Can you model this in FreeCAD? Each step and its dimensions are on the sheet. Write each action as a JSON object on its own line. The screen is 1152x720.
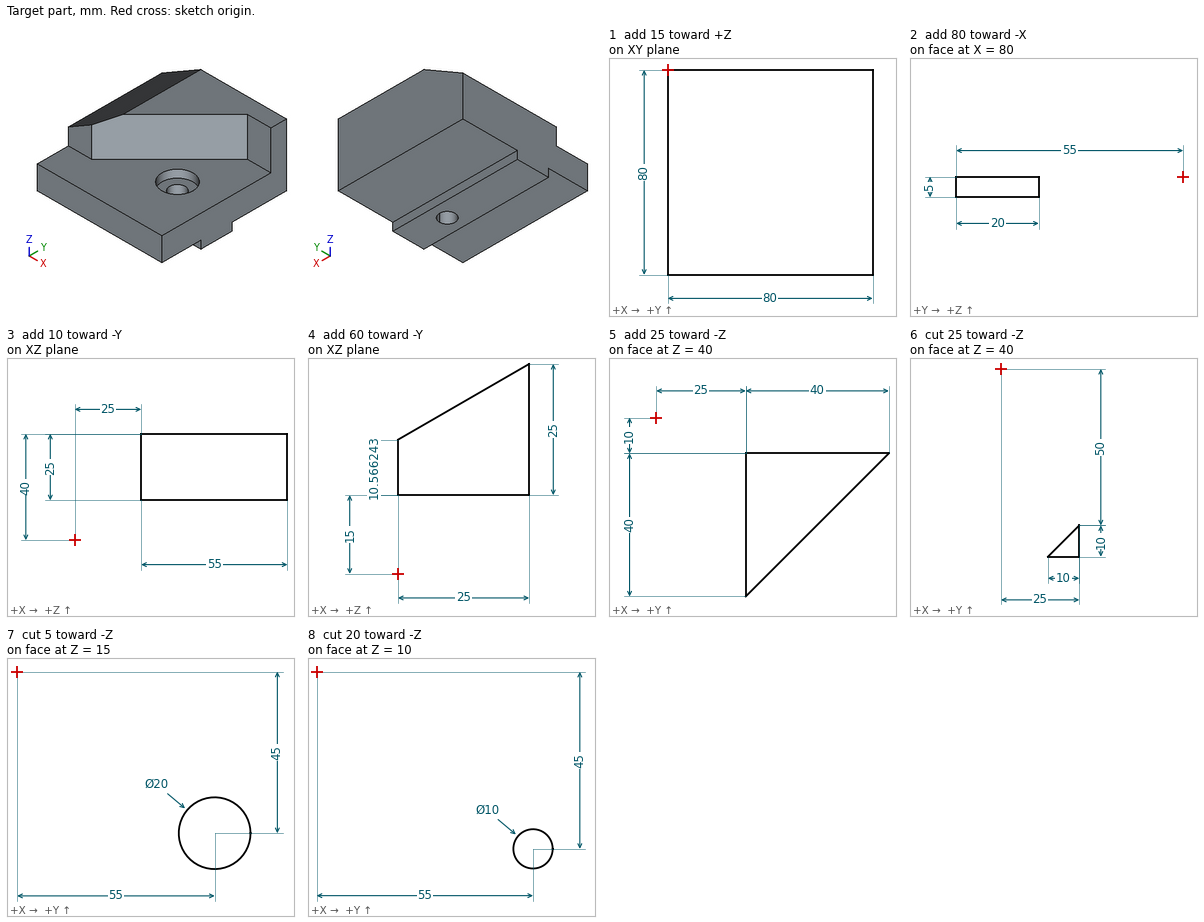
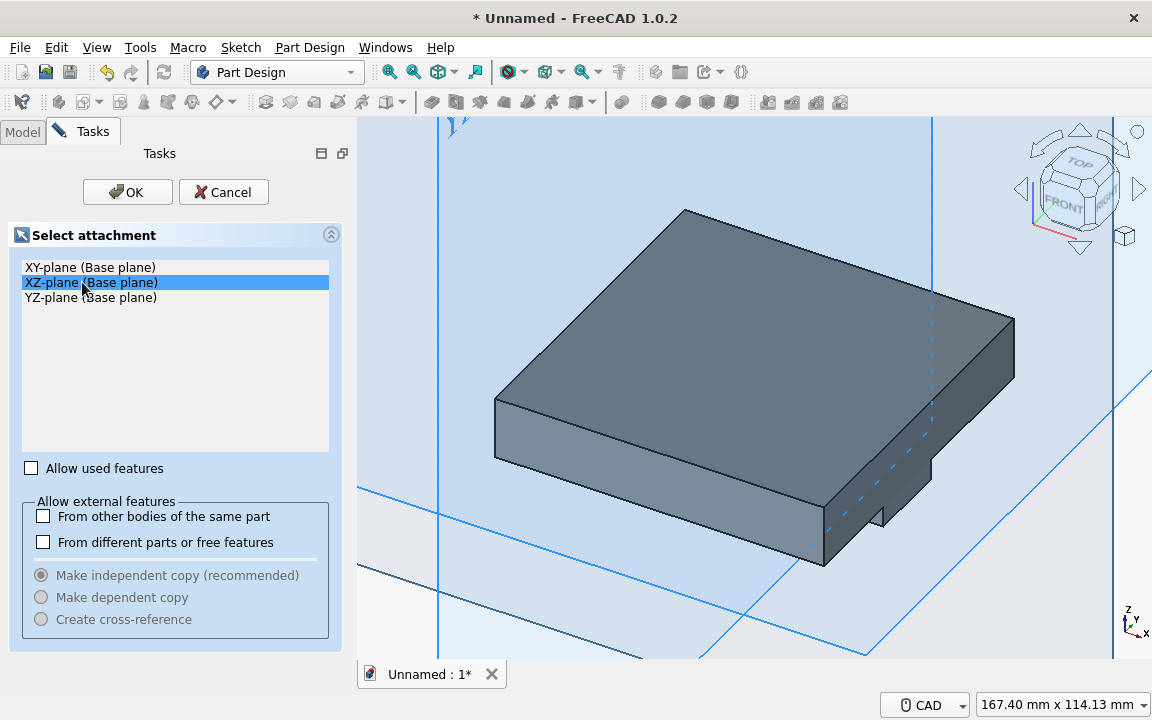
{"action": "left_click", "coordinate": [128, 192]}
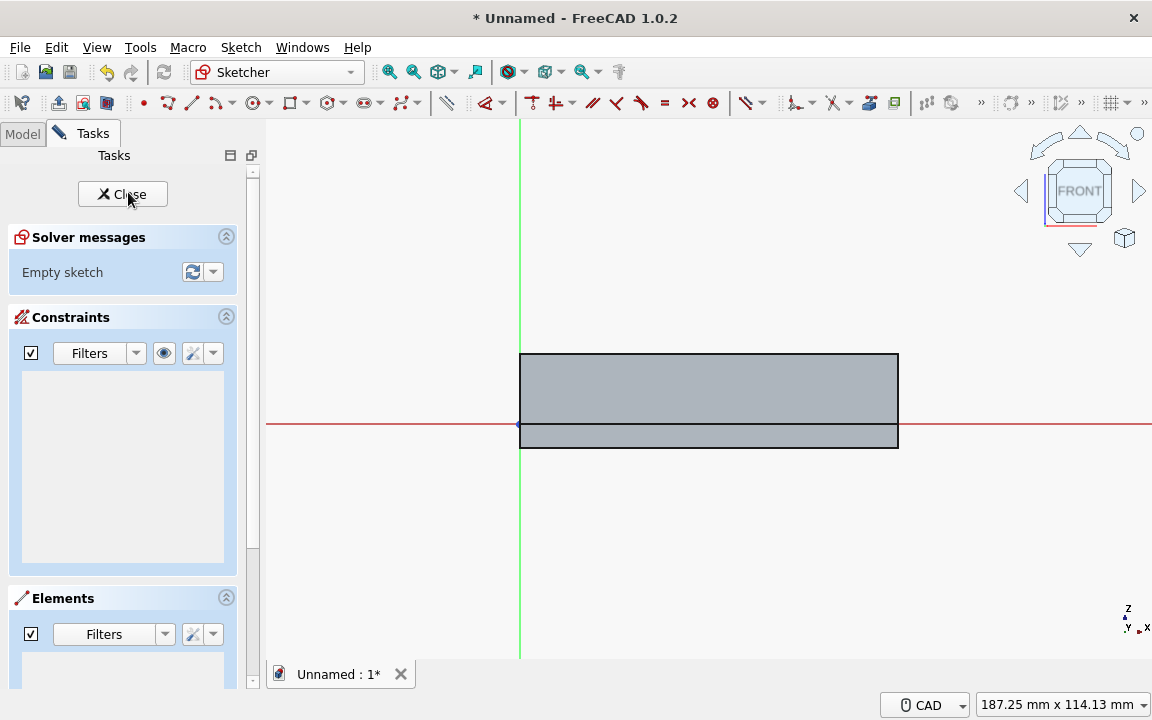
{"action": "left_click", "coordinate": [108, 104]}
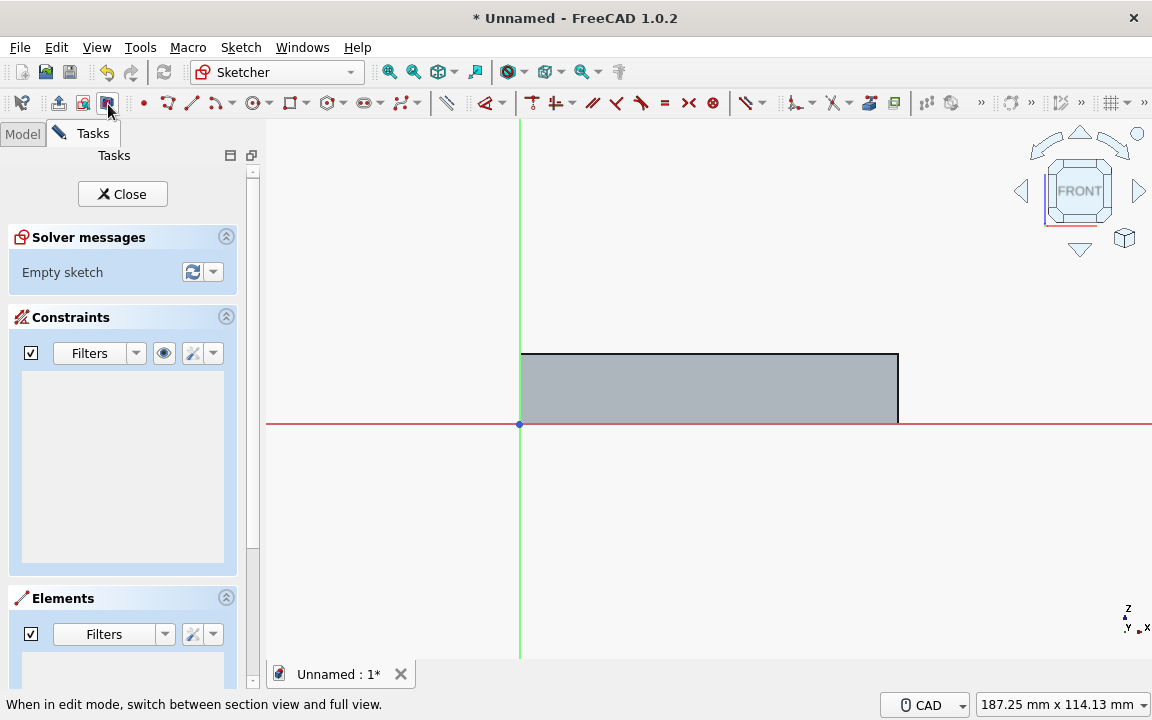
{"action": "left_click", "coordinate": [290, 104]}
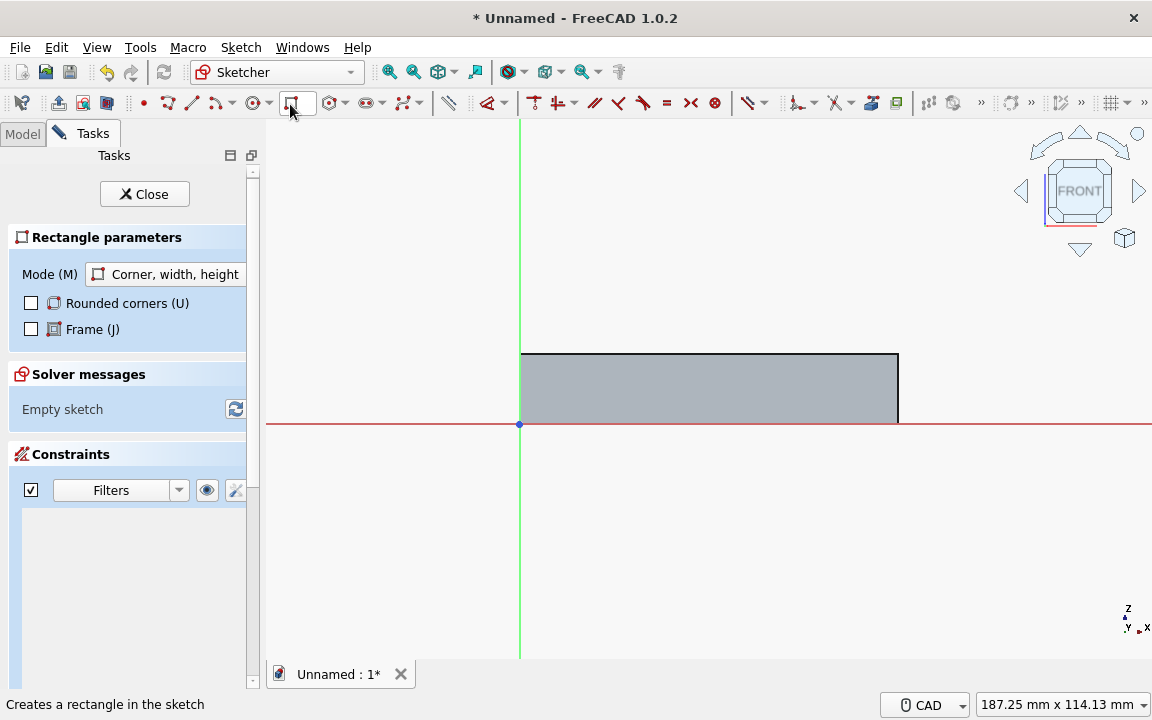
{"action": "left_click", "coordinate": [638, 235]}
{"action": "left_click", "coordinate": [898, 354]}
{"action": "key", "text": "Escape"}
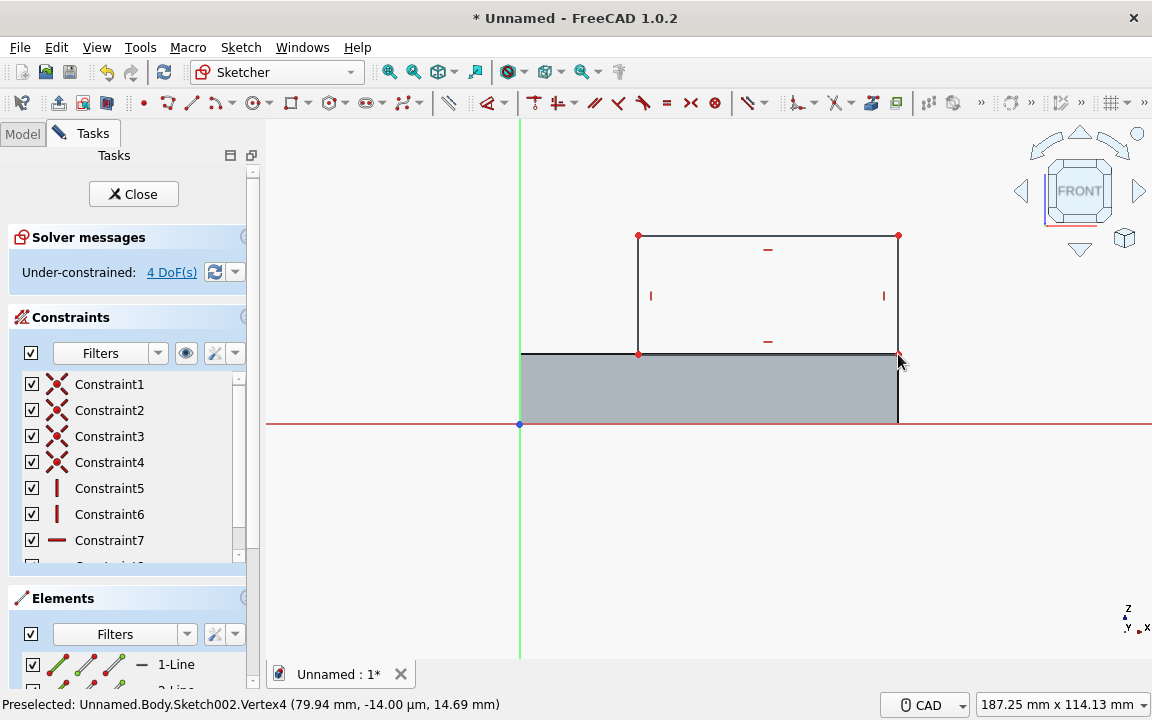
{"action": "left_click", "coordinate": [488, 104]}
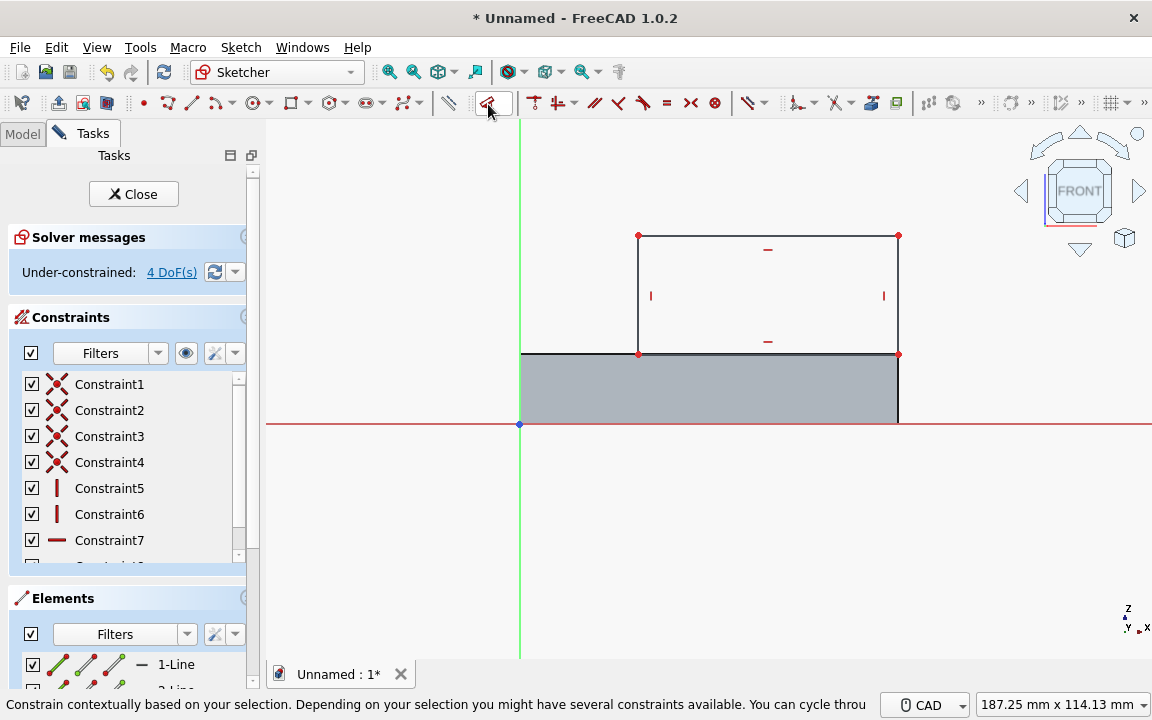
{"action": "left_click", "coordinate": [638, 272]}
{"action": "left_click", "coordinate": [604, 295]}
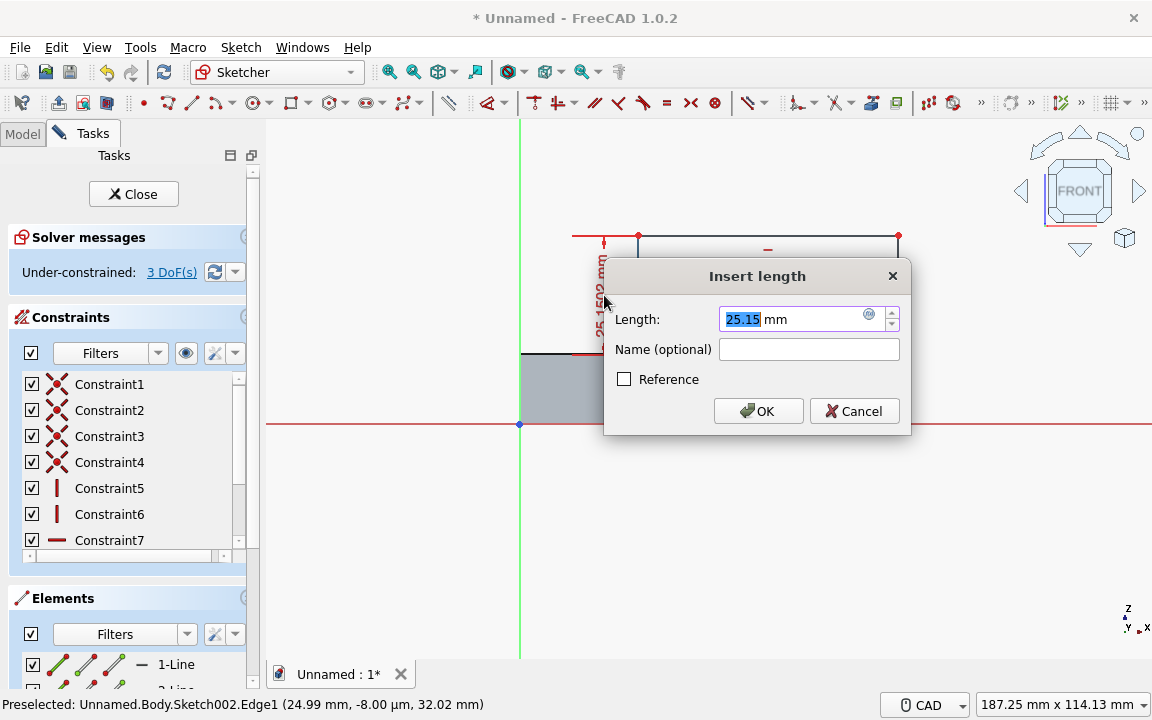
{"action": "type", "text": "25"}
{"action": "key", "text": "Return"}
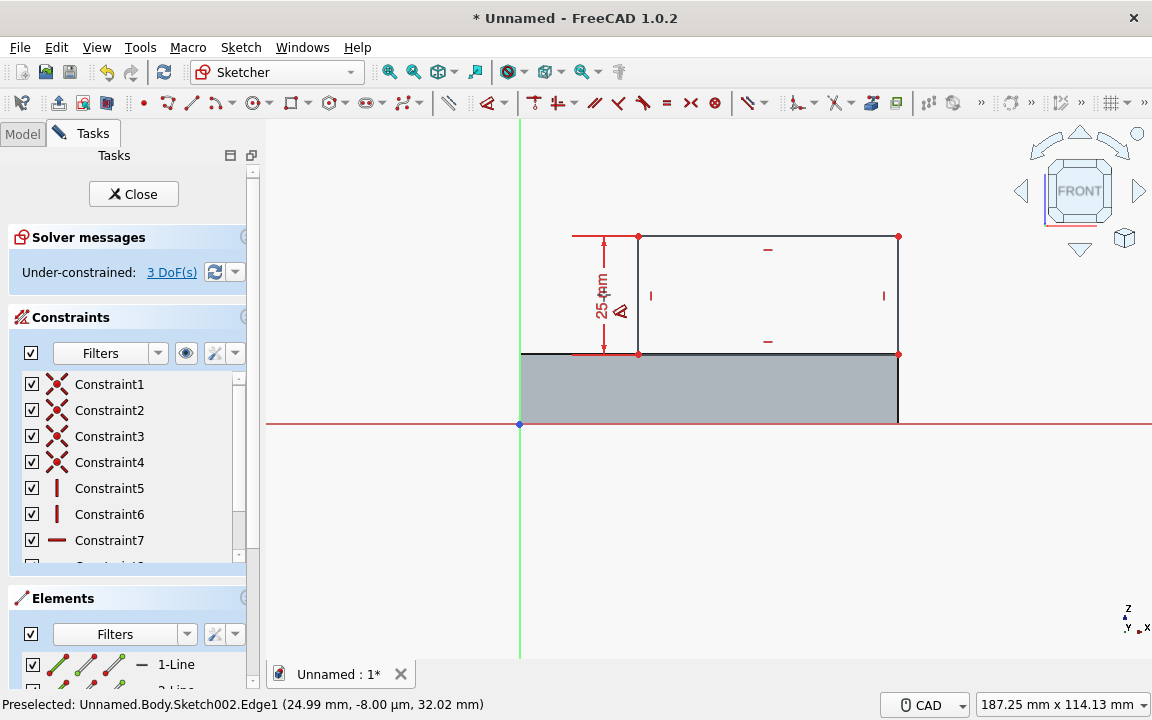
{"action": "left_click", "coordinate": [716, 355]}
{"action": "left_click", "coordinate": [768, 389]}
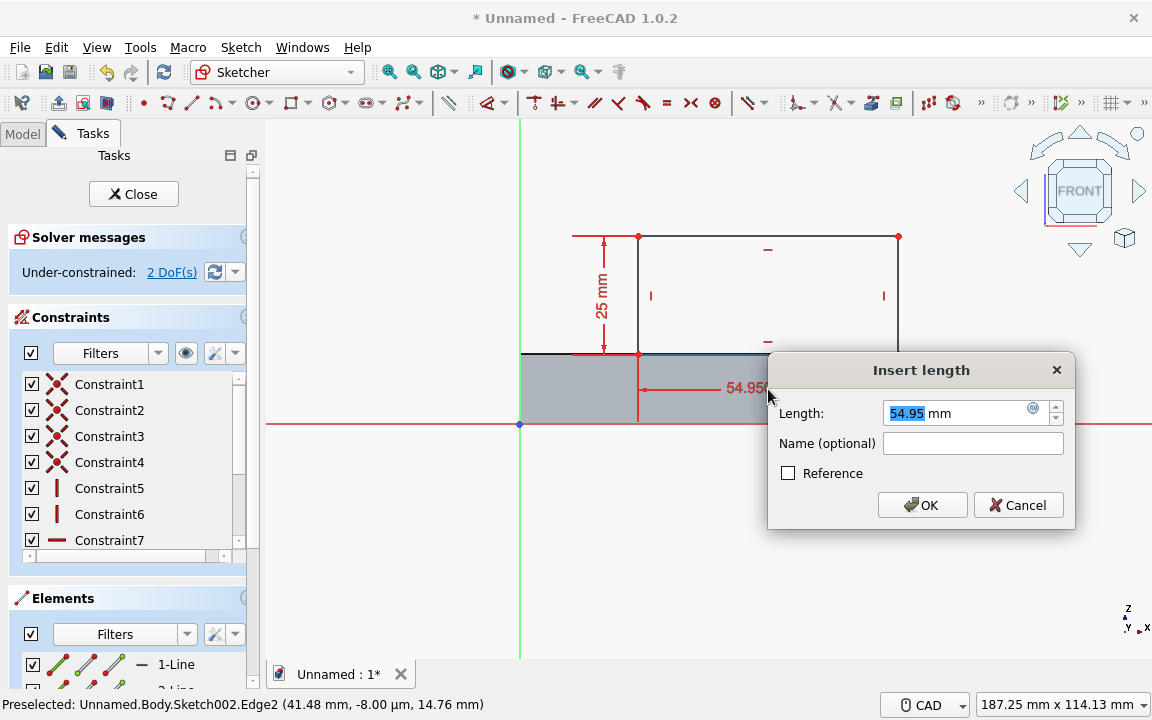
{"action": "type", "text": "55"}
{"action": "key", "text": "Return"}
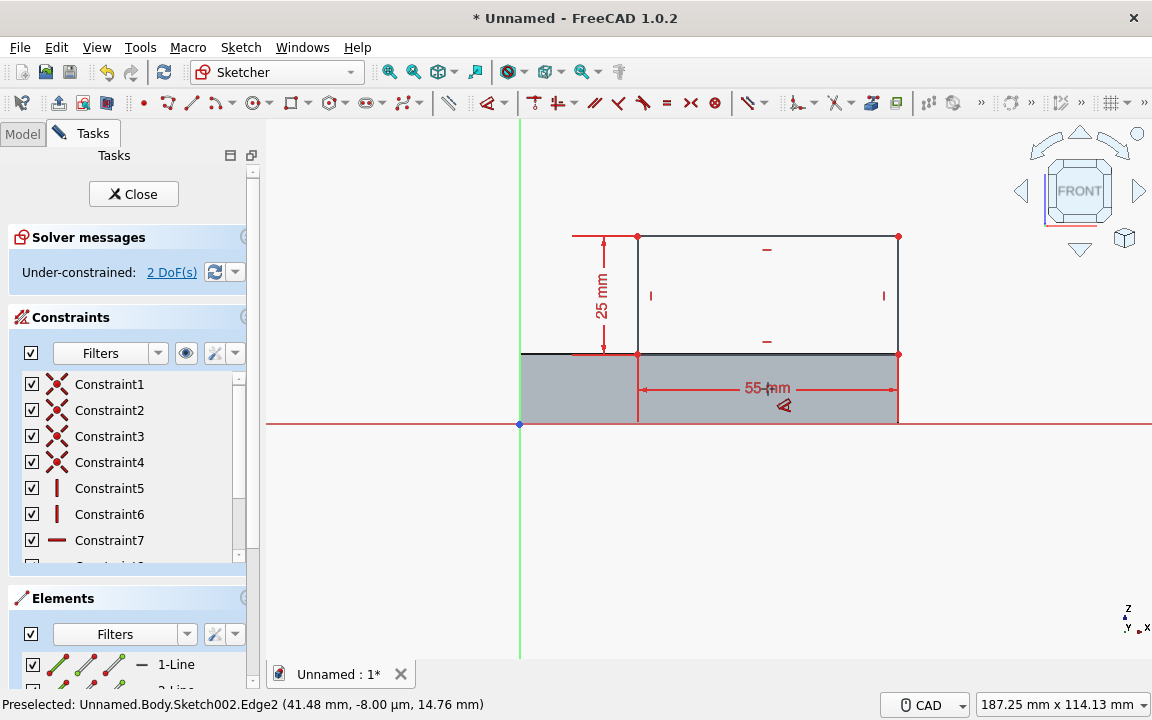
{"action": "left_click", "coordinate": [638, 236]}
{"action": "left_click", "coordinate": [579, 458]}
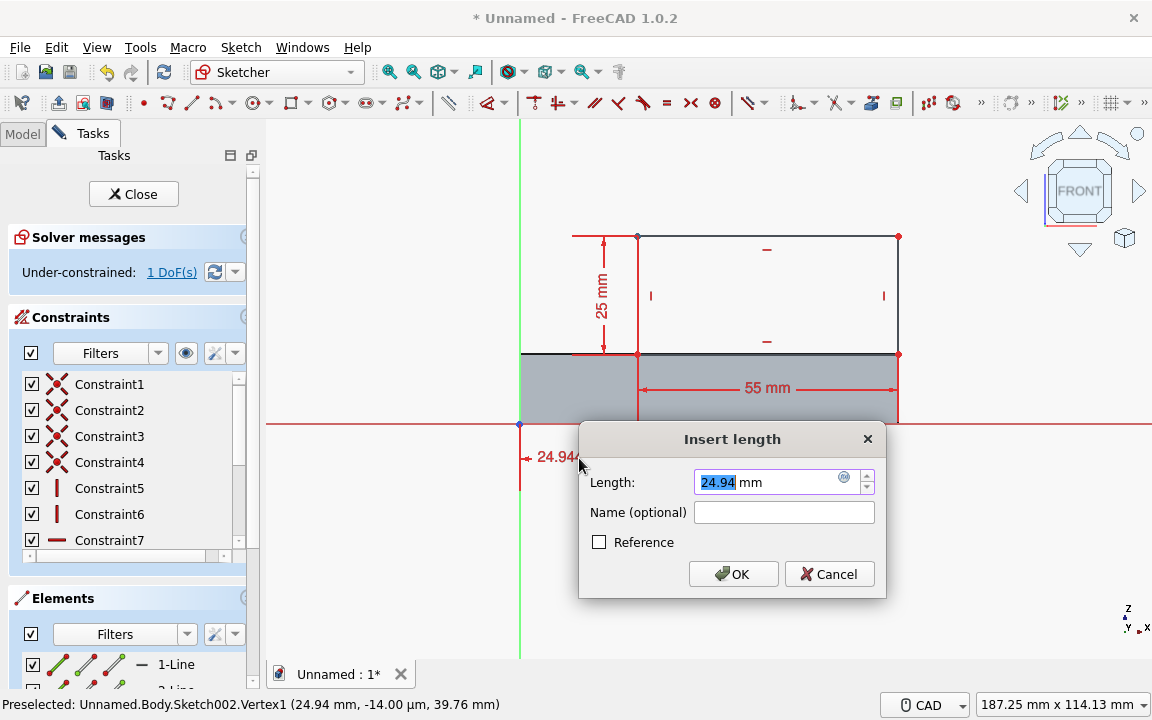
{"action": "type", "text": "25"}
{"action": "key", "text": "Return"}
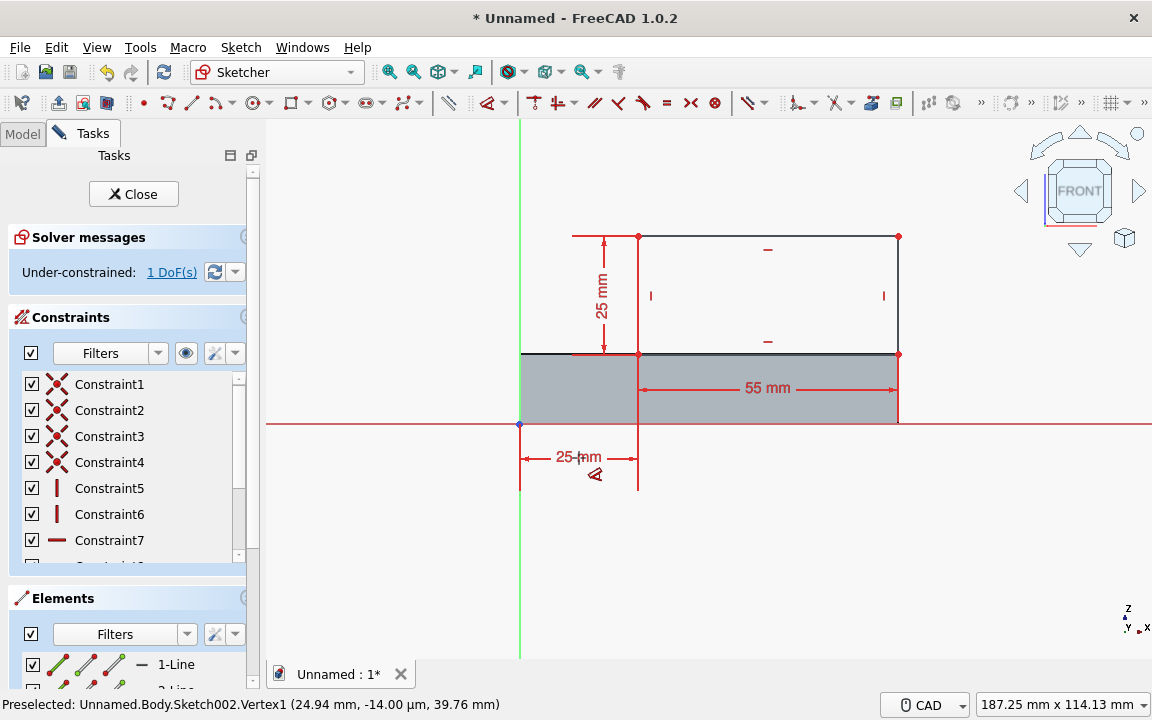
{"action": "left_click", "coordinate": [638, 236]}
{"action": "left_click", "coordinate": [486, 330]}